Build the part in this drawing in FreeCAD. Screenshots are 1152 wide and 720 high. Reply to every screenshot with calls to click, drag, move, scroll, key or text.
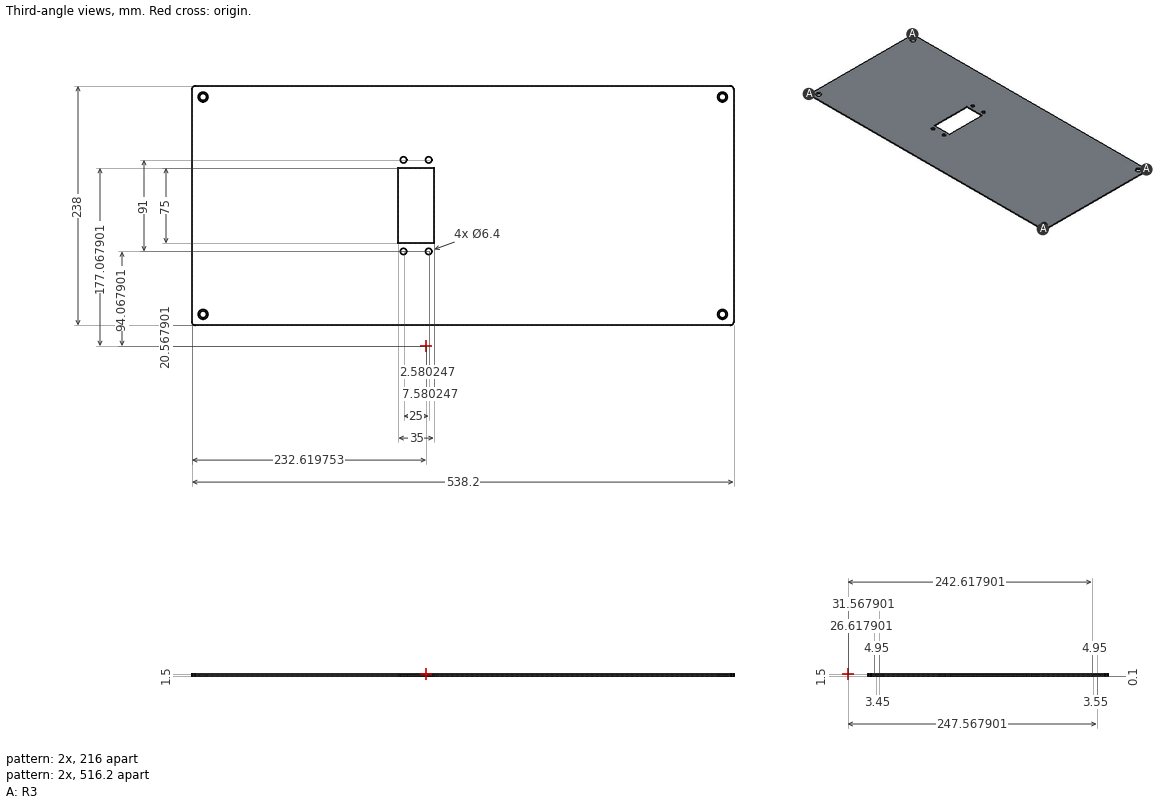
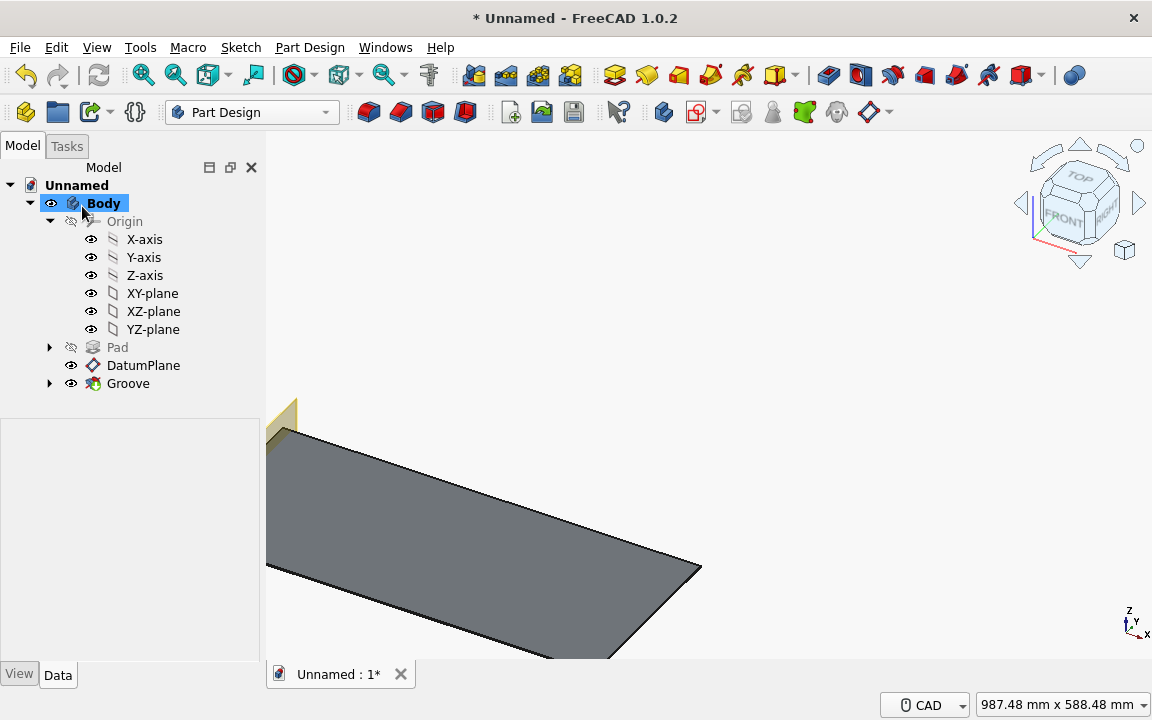
click(116, 365)
key(space)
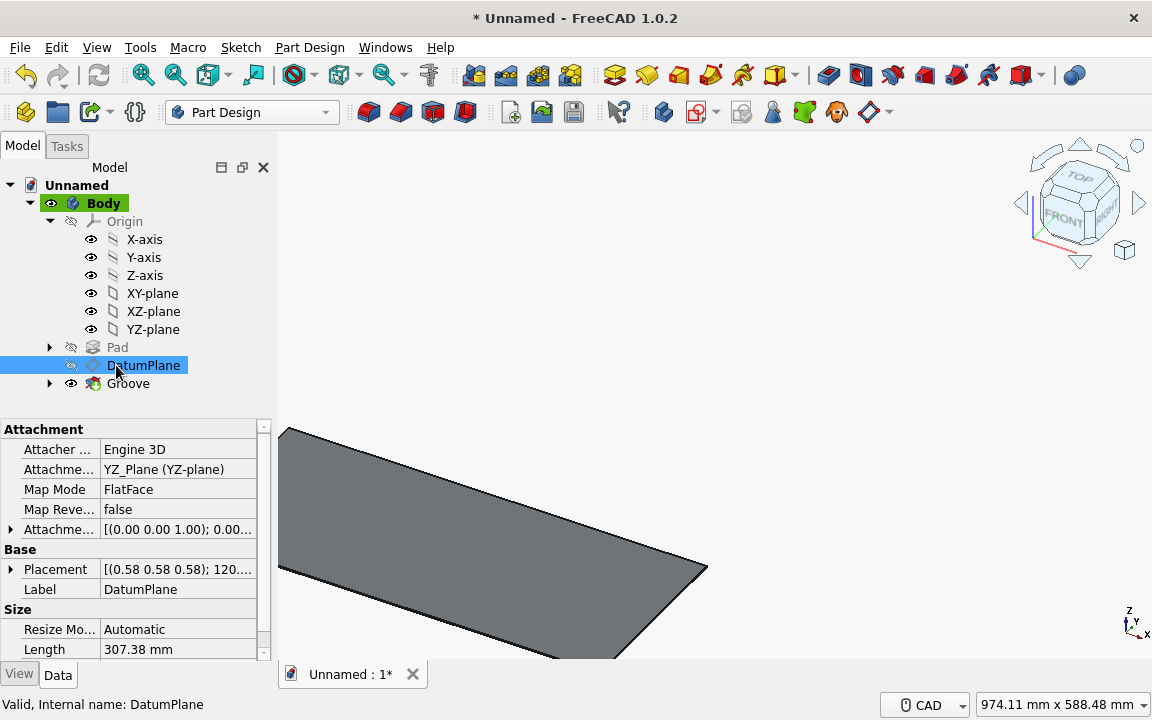
click(144, 76)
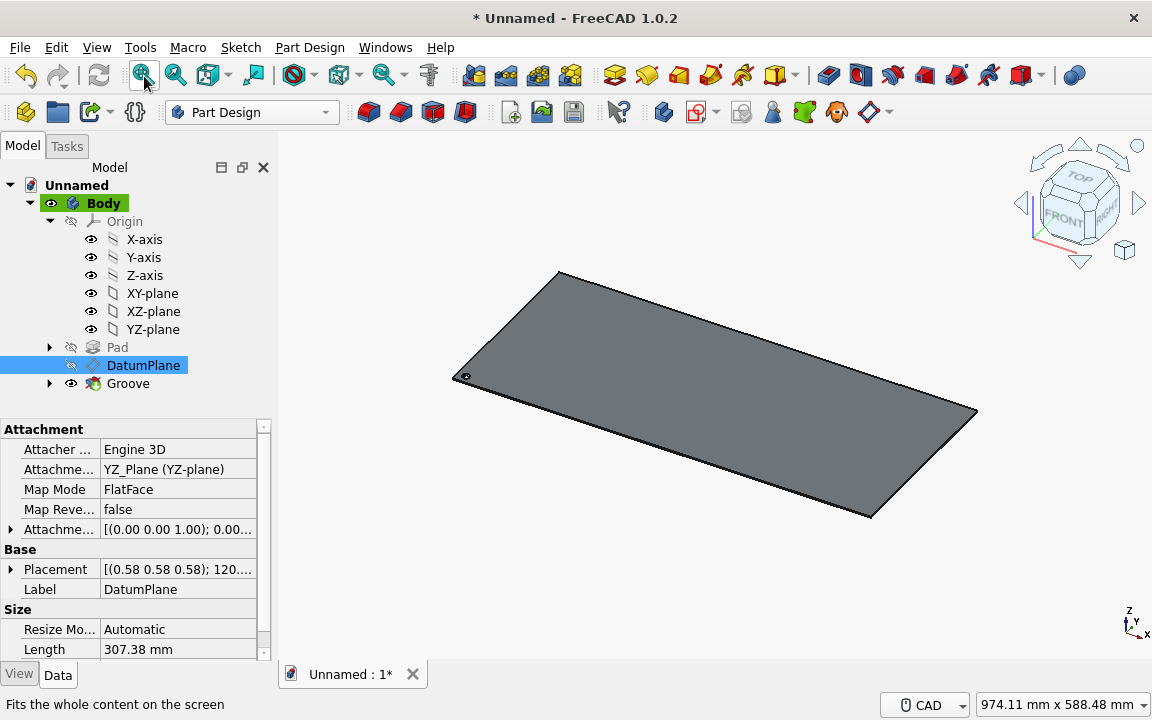
click(136, 329)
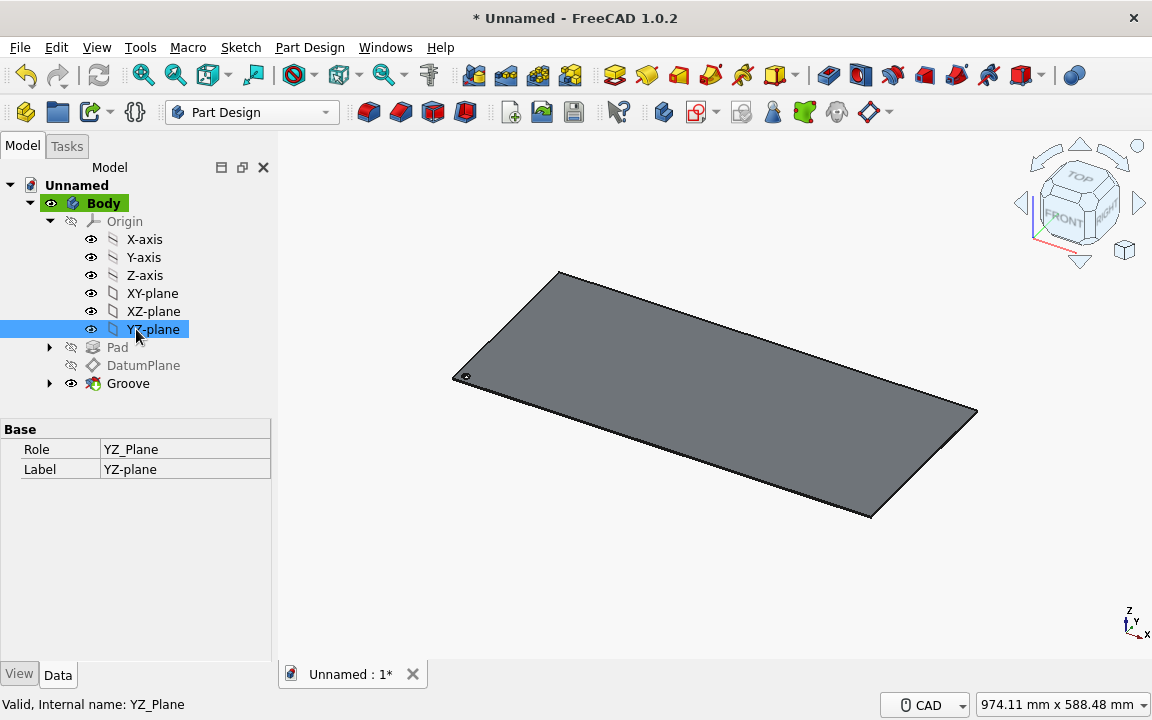
click(870, 112)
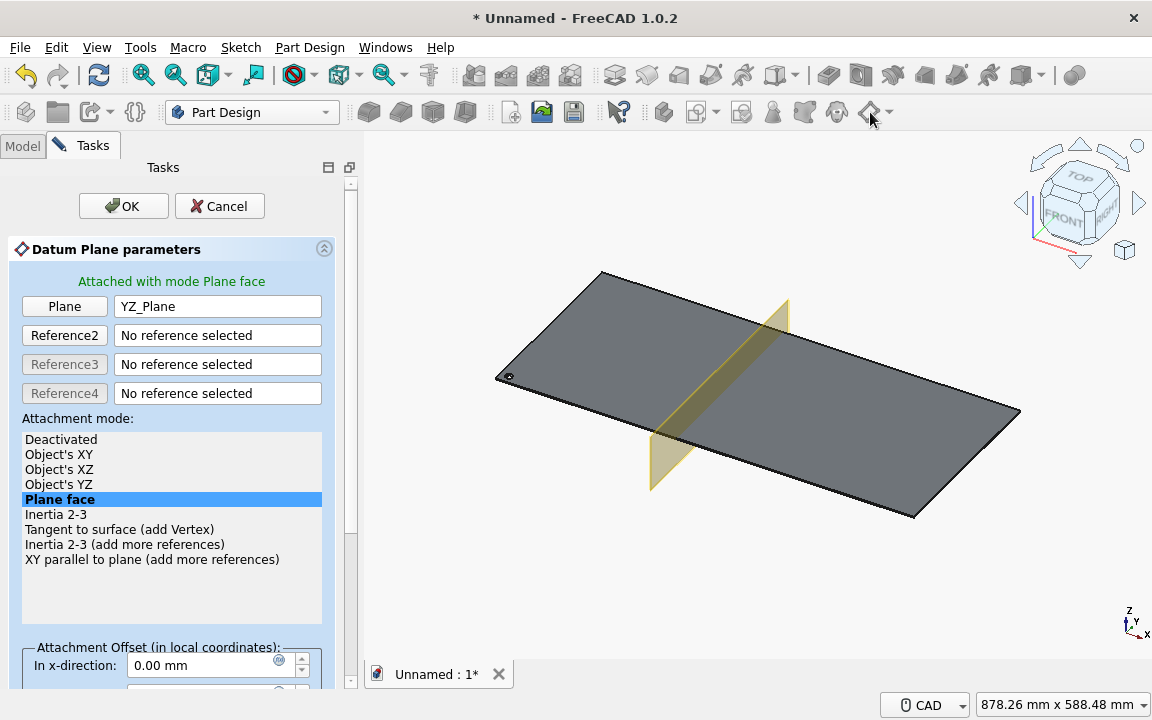
scroll(351, 432, down, 2)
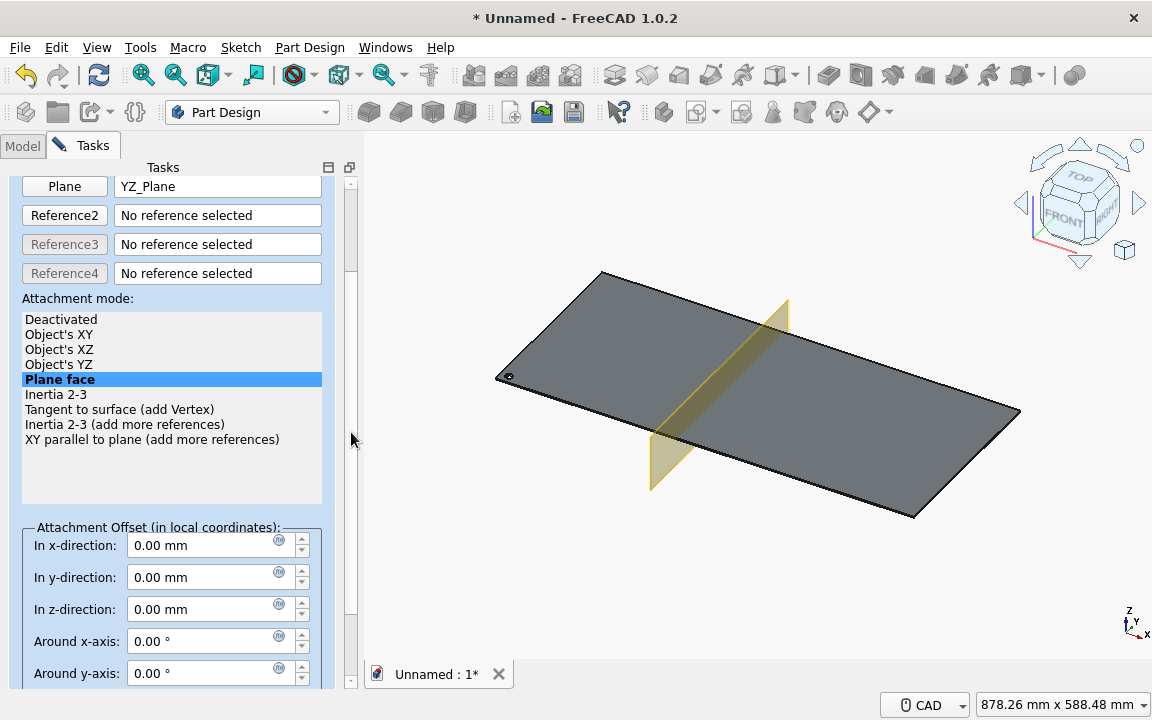
triple_click(210, 609)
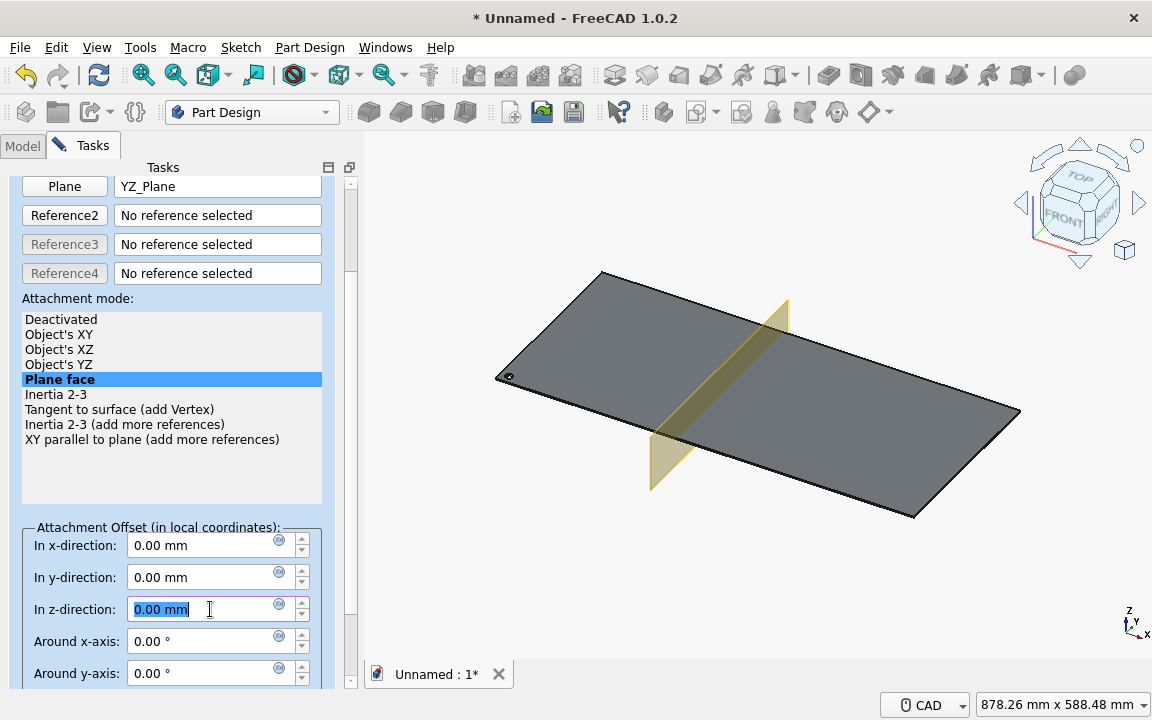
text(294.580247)
key(Tab)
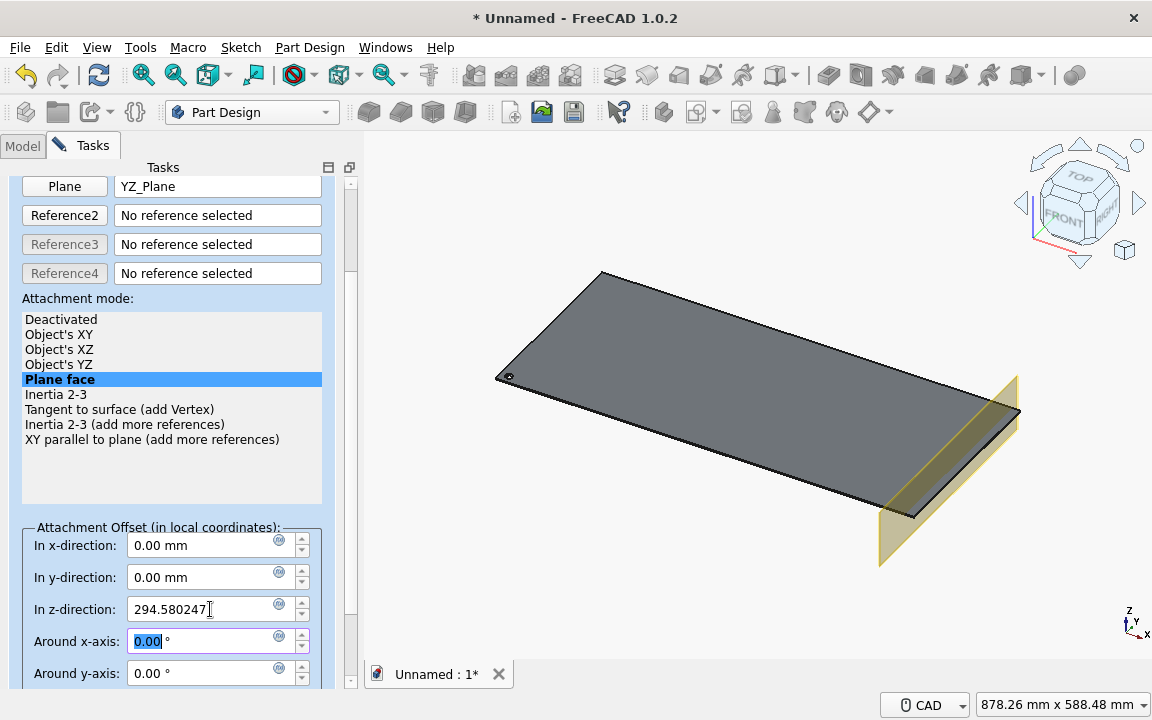
scroll(351, 432, up, 3)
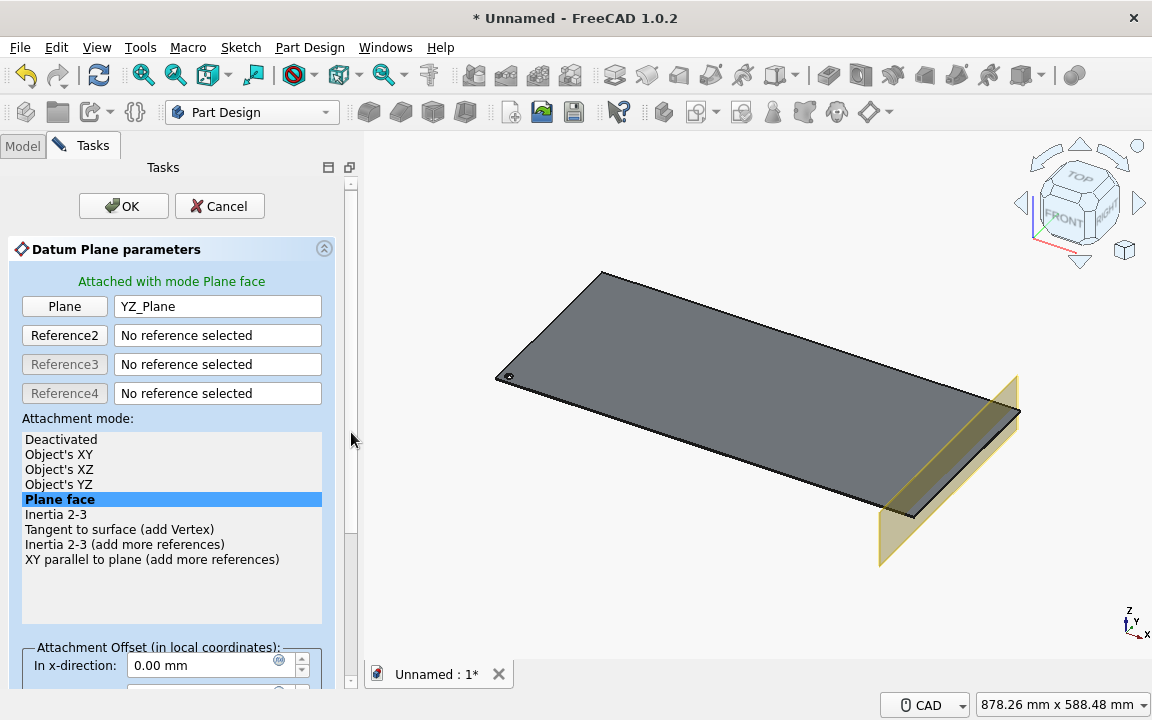
click(124, 206)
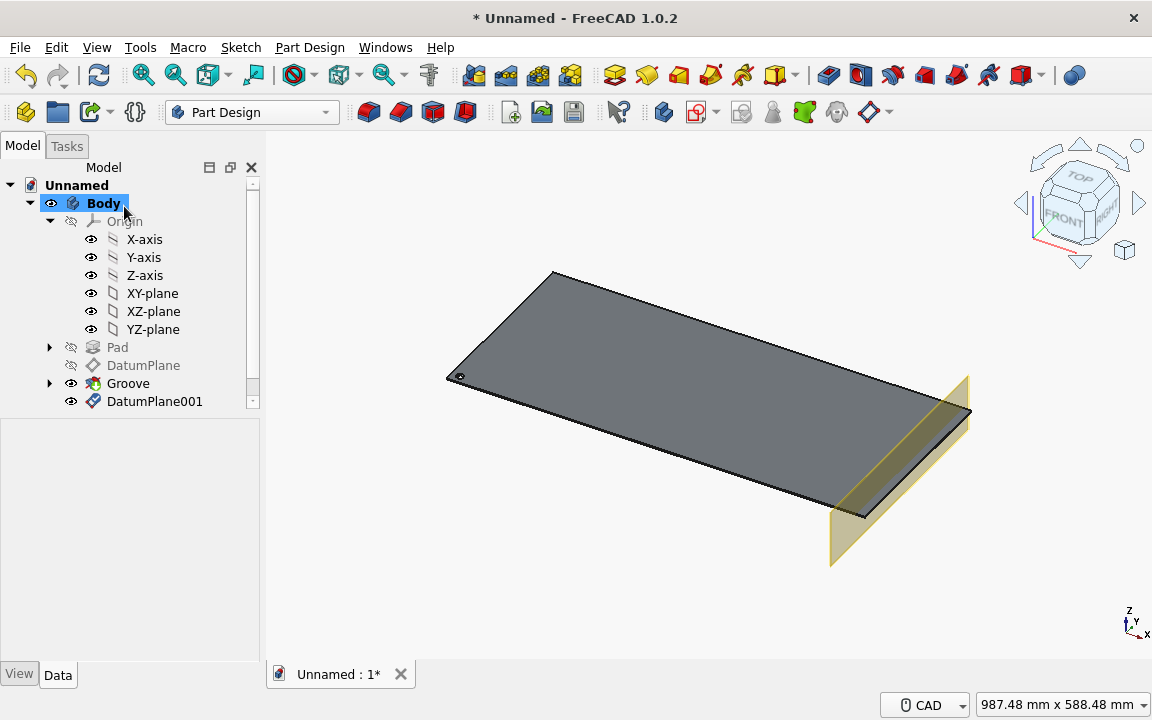
click(116, 401)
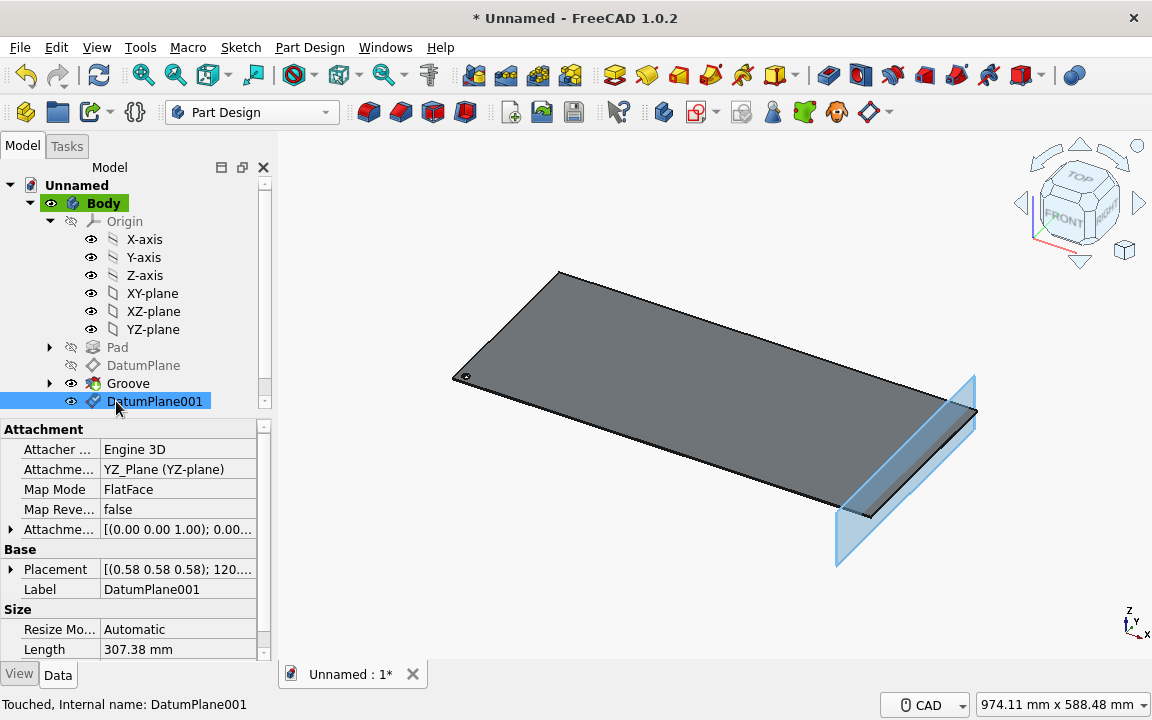
click(696, 112)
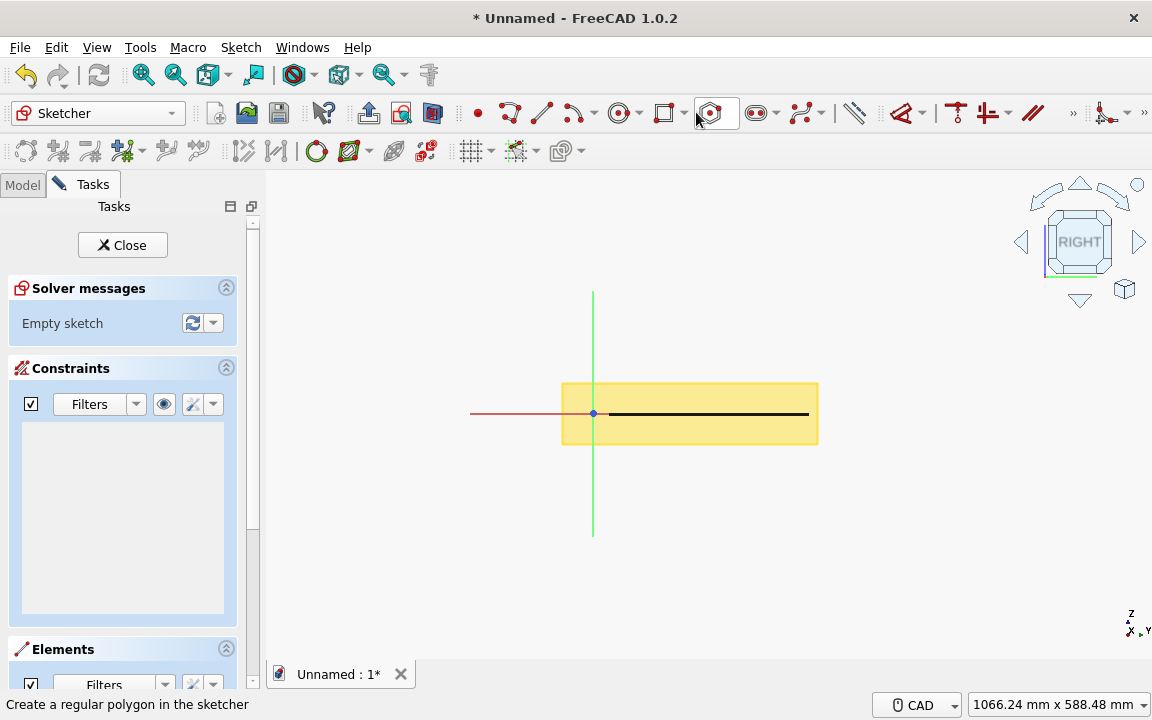
click(434, 114)